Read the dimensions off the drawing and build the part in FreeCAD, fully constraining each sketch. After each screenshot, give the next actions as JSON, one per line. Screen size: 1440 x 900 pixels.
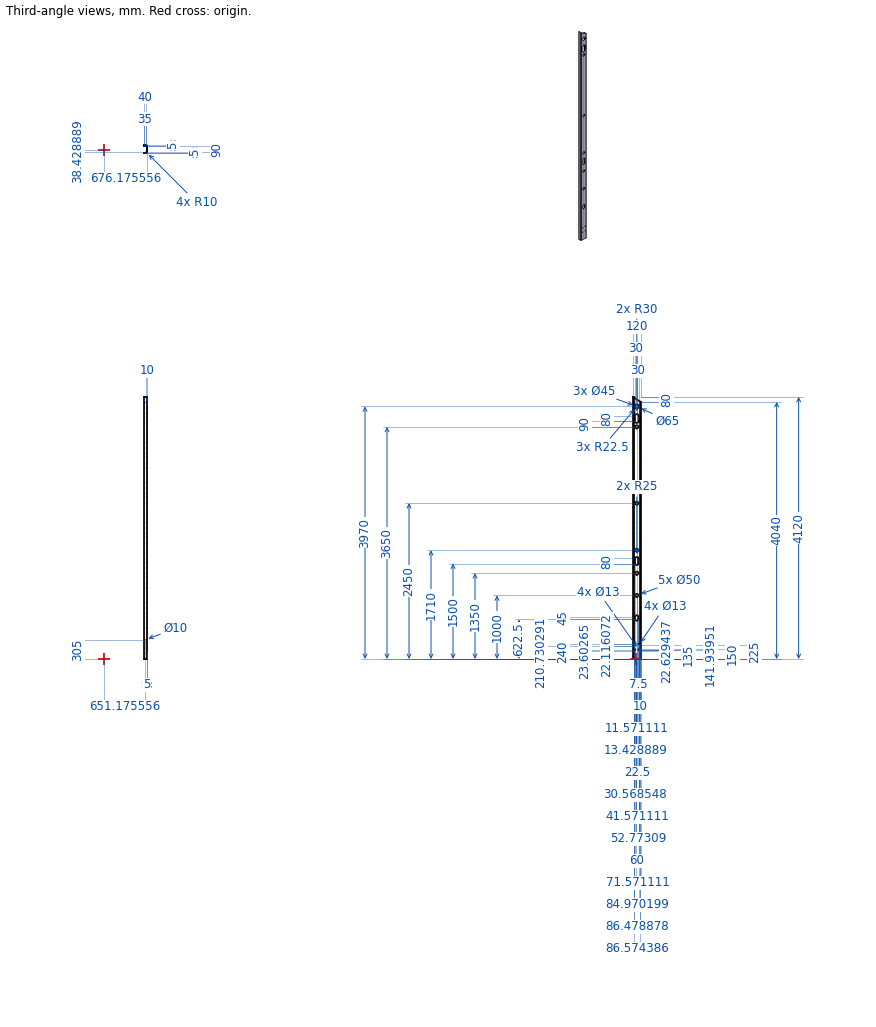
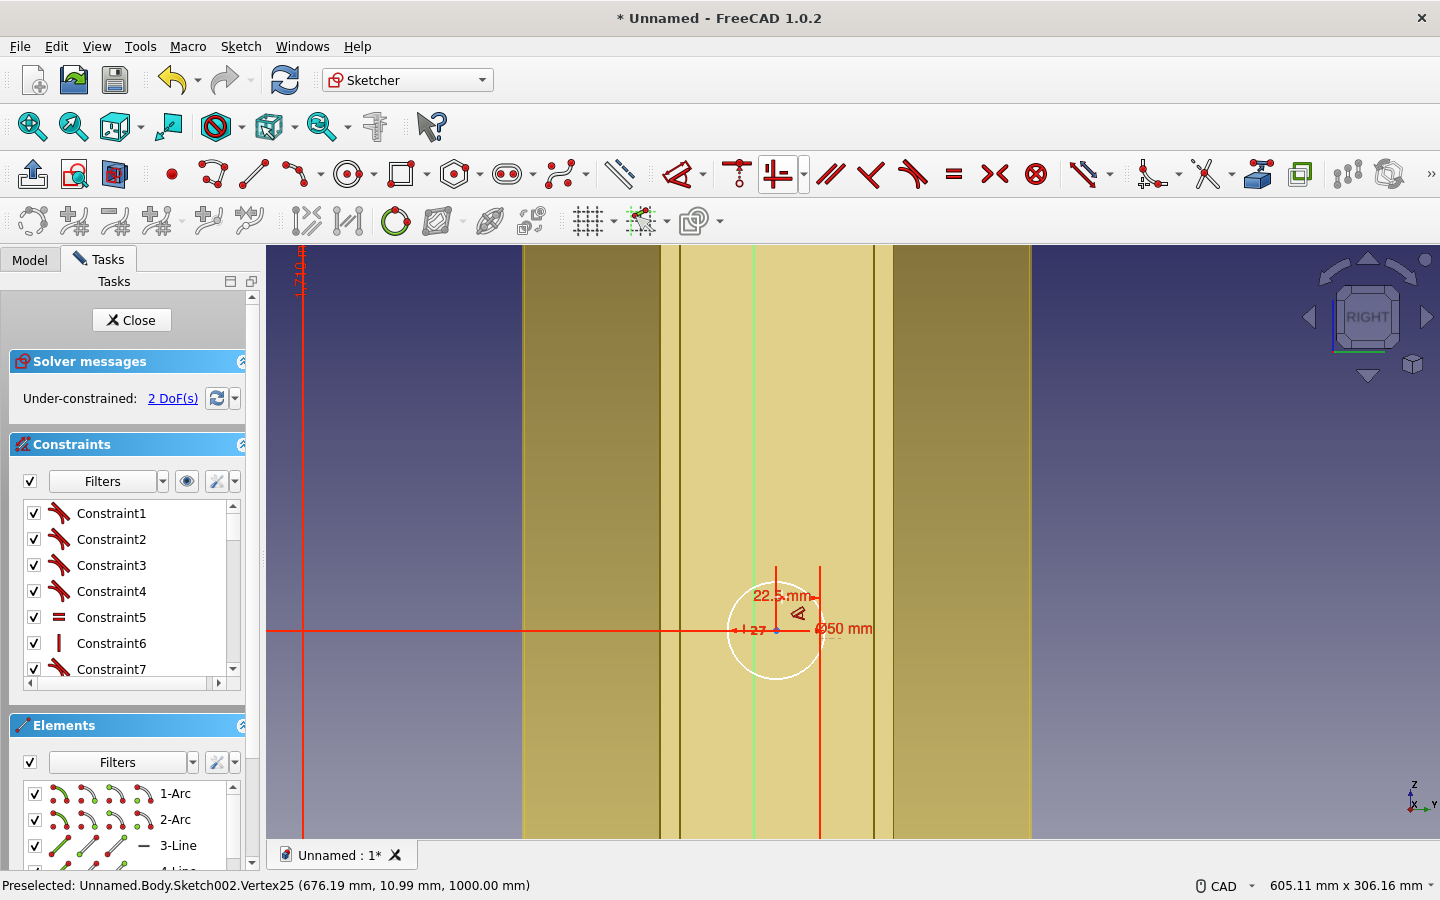
{"action": "scroll", "coordinate": [785, 639], "scroll_direction": "down", "scroll_amount": 15}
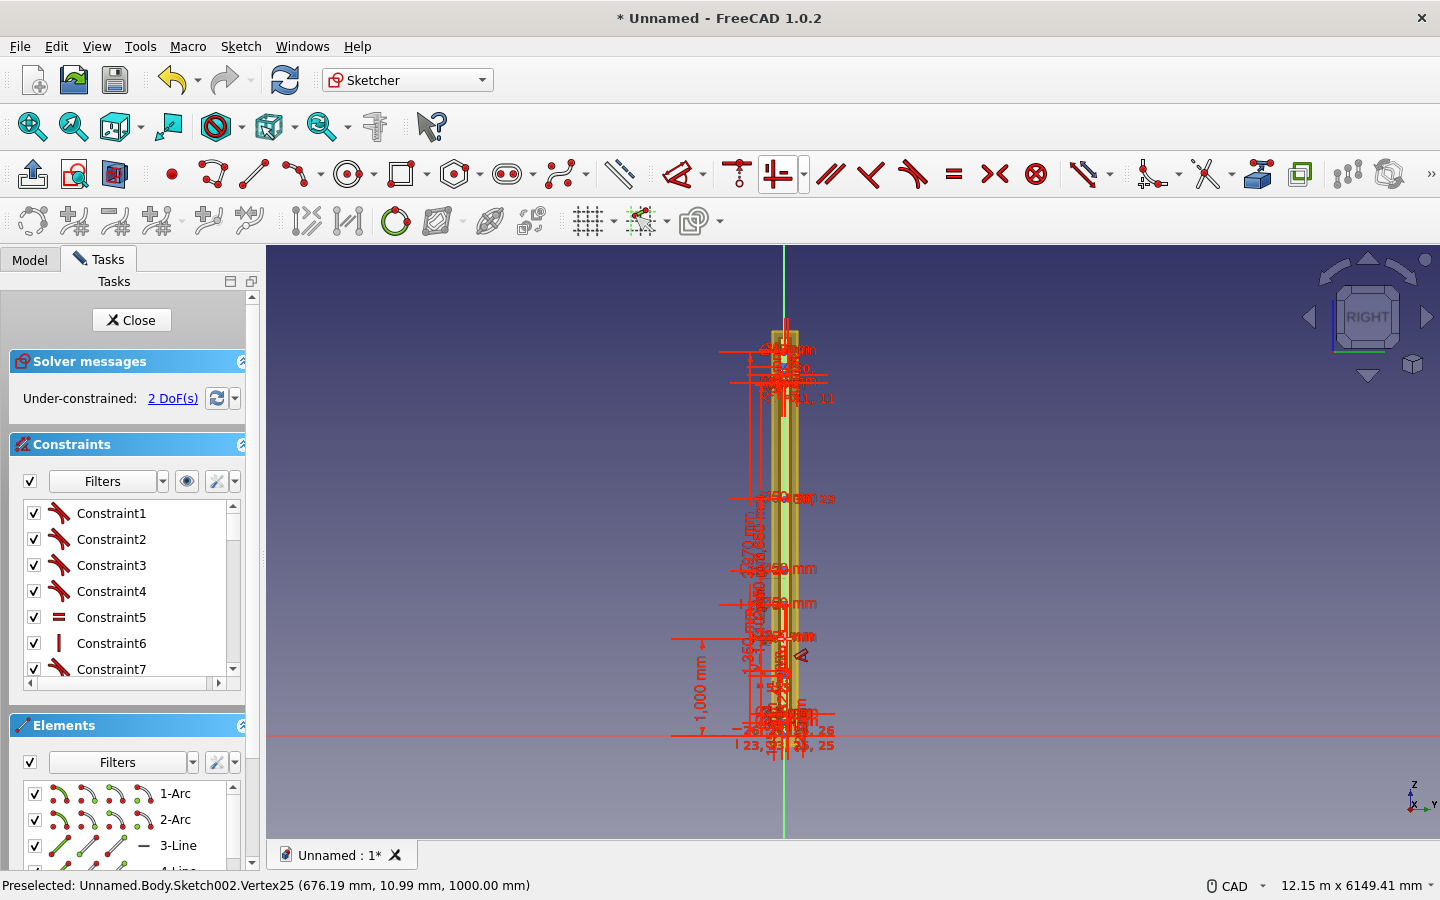
{"action": "scroll", "coordinate": [783, 676], "scroll_direction": "up", "scroll_amount": 9}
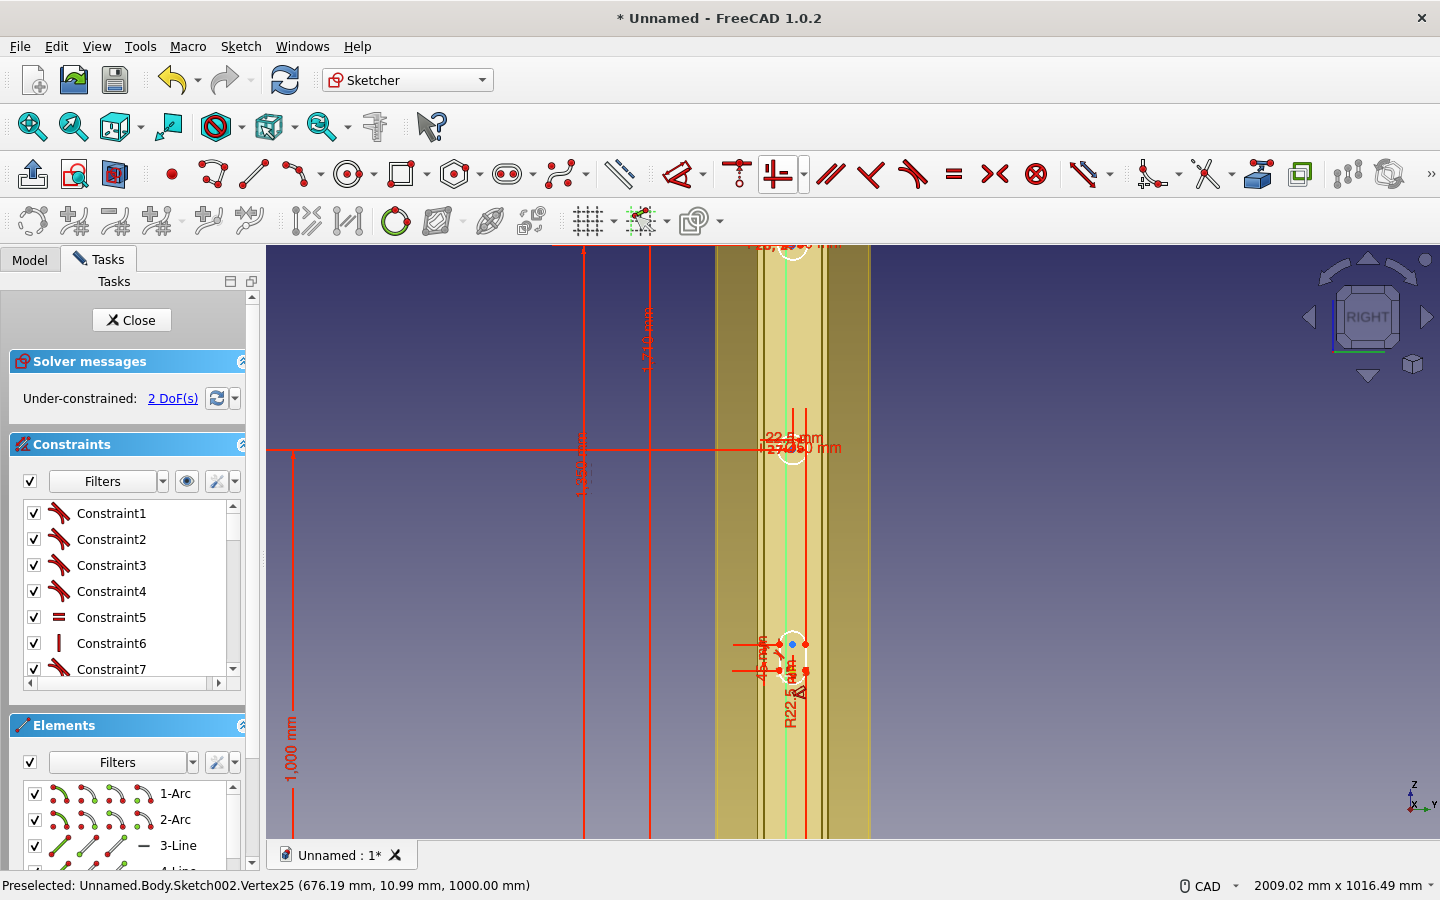
{"action": "left_click", "coordinate": [780, 671]}
{"action": "left_click", "coordinate": [746, 741]}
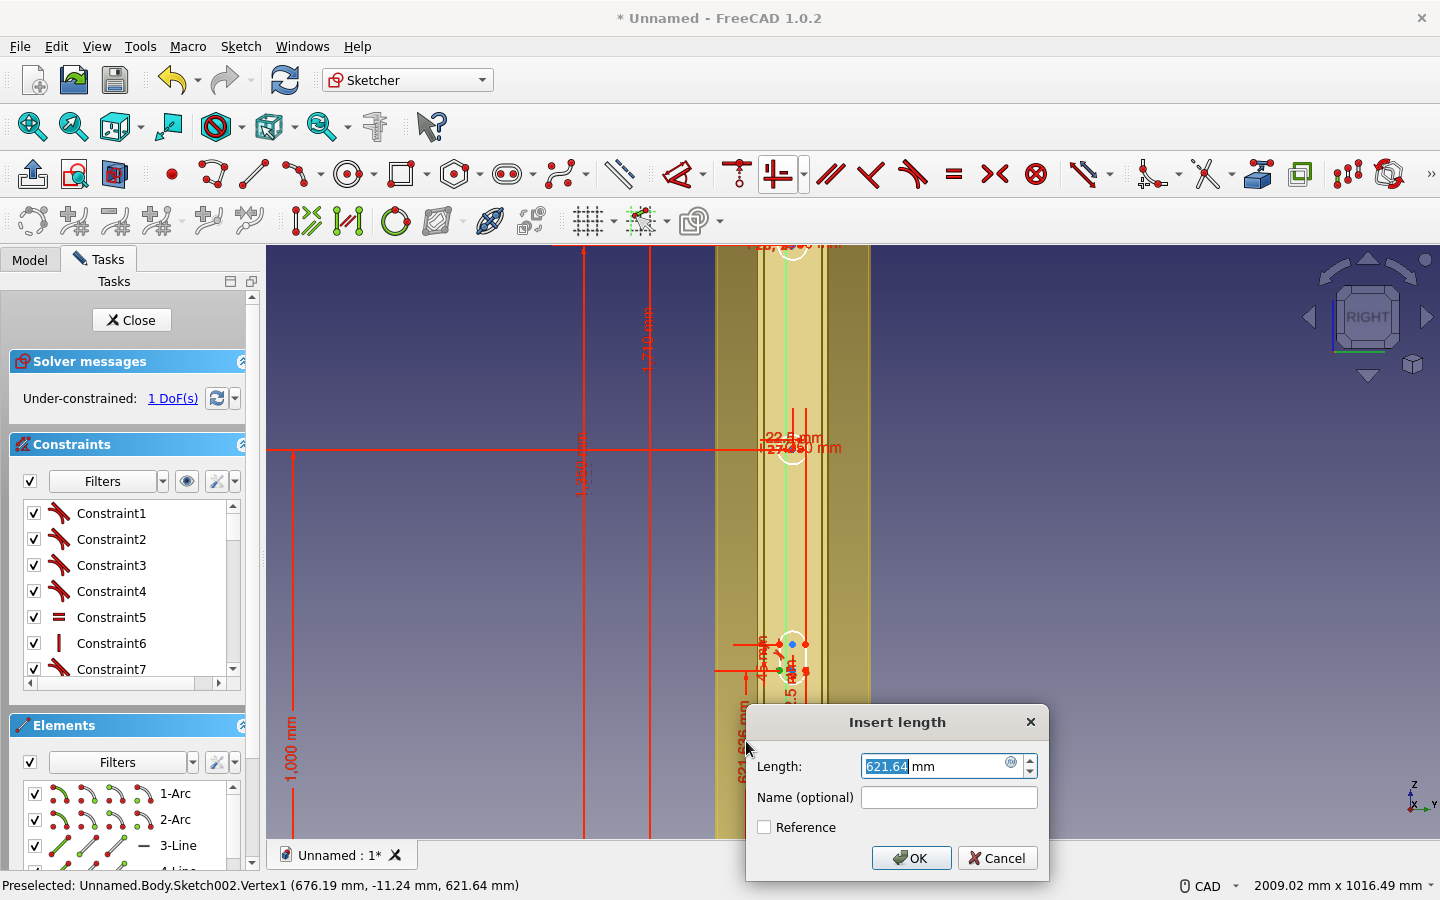
{"action": "type", "text": "622.5"}
{"action": "key", "text": "Return"}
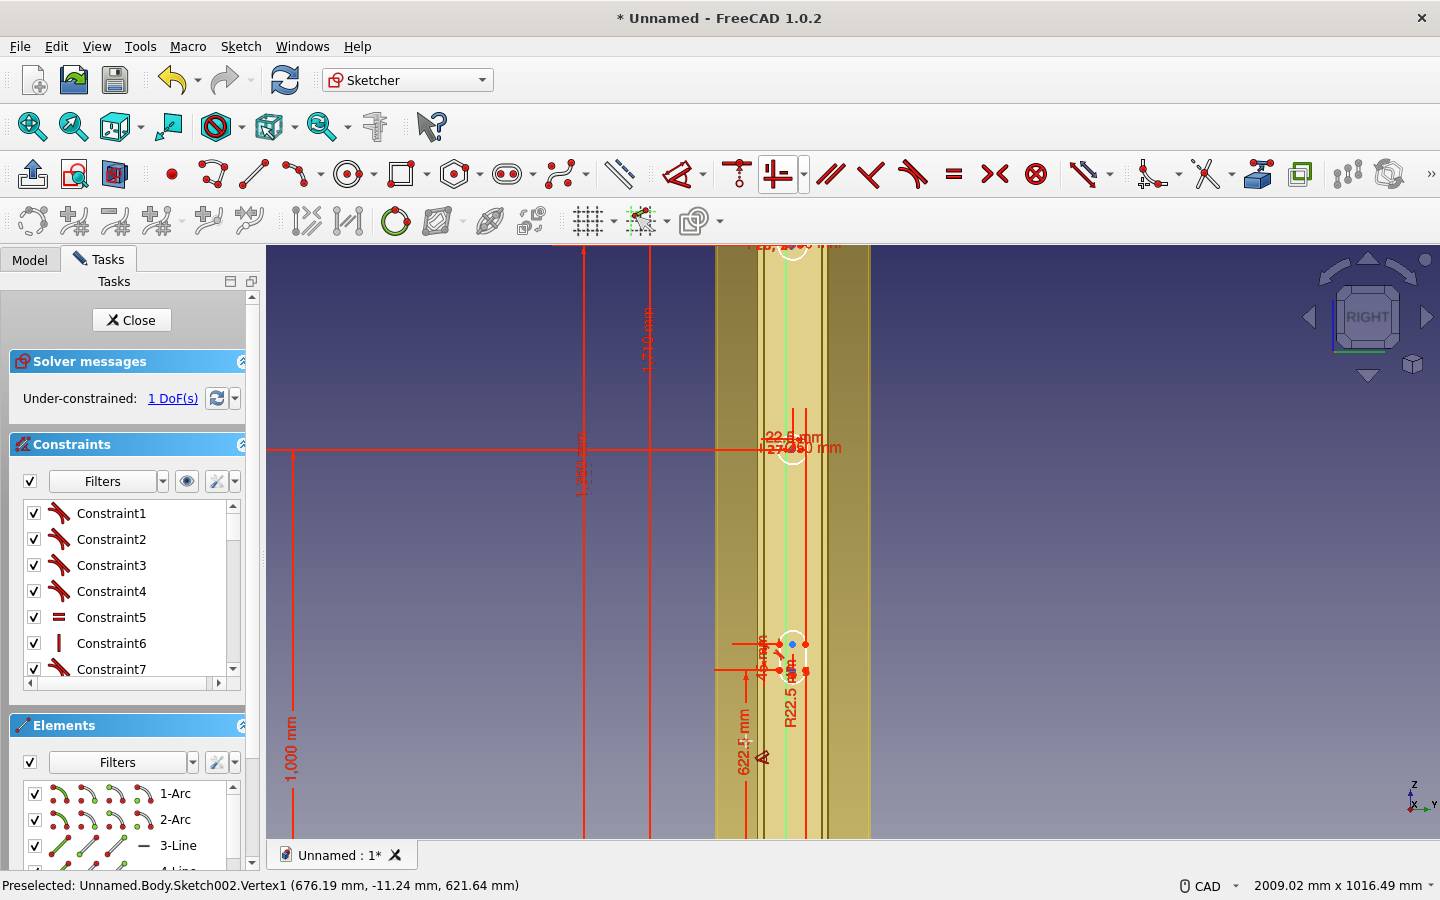
{"action": "scroll", "coordinate": [783, 676], "scroll_direction": "down", "scroll_amount": 9}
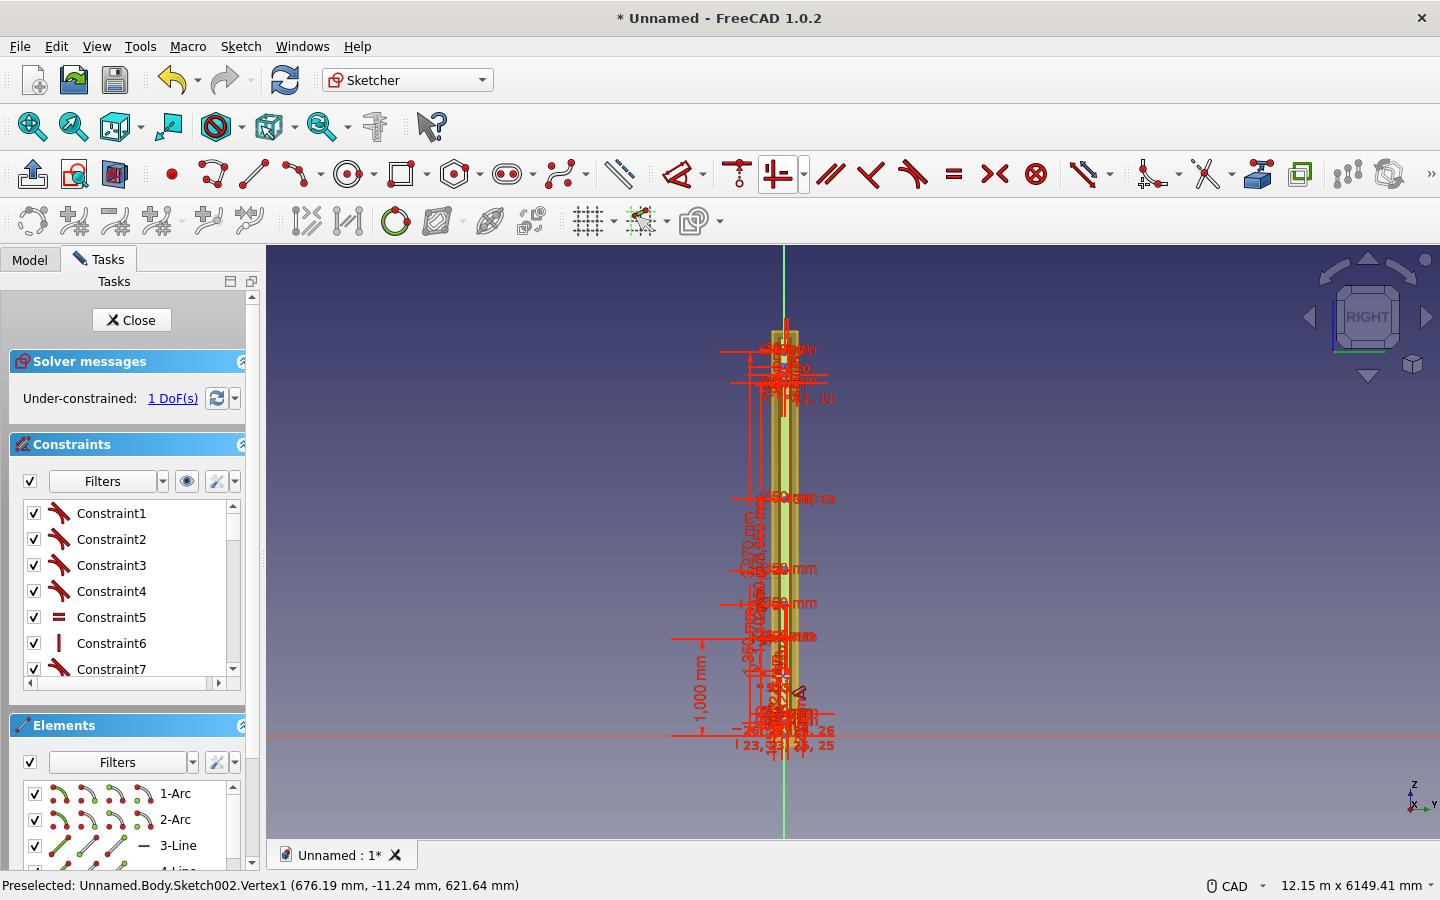
{"action": "scroll", "coordinate": [788, 714], "scroll_direction": "up", "scroll_amount": 12}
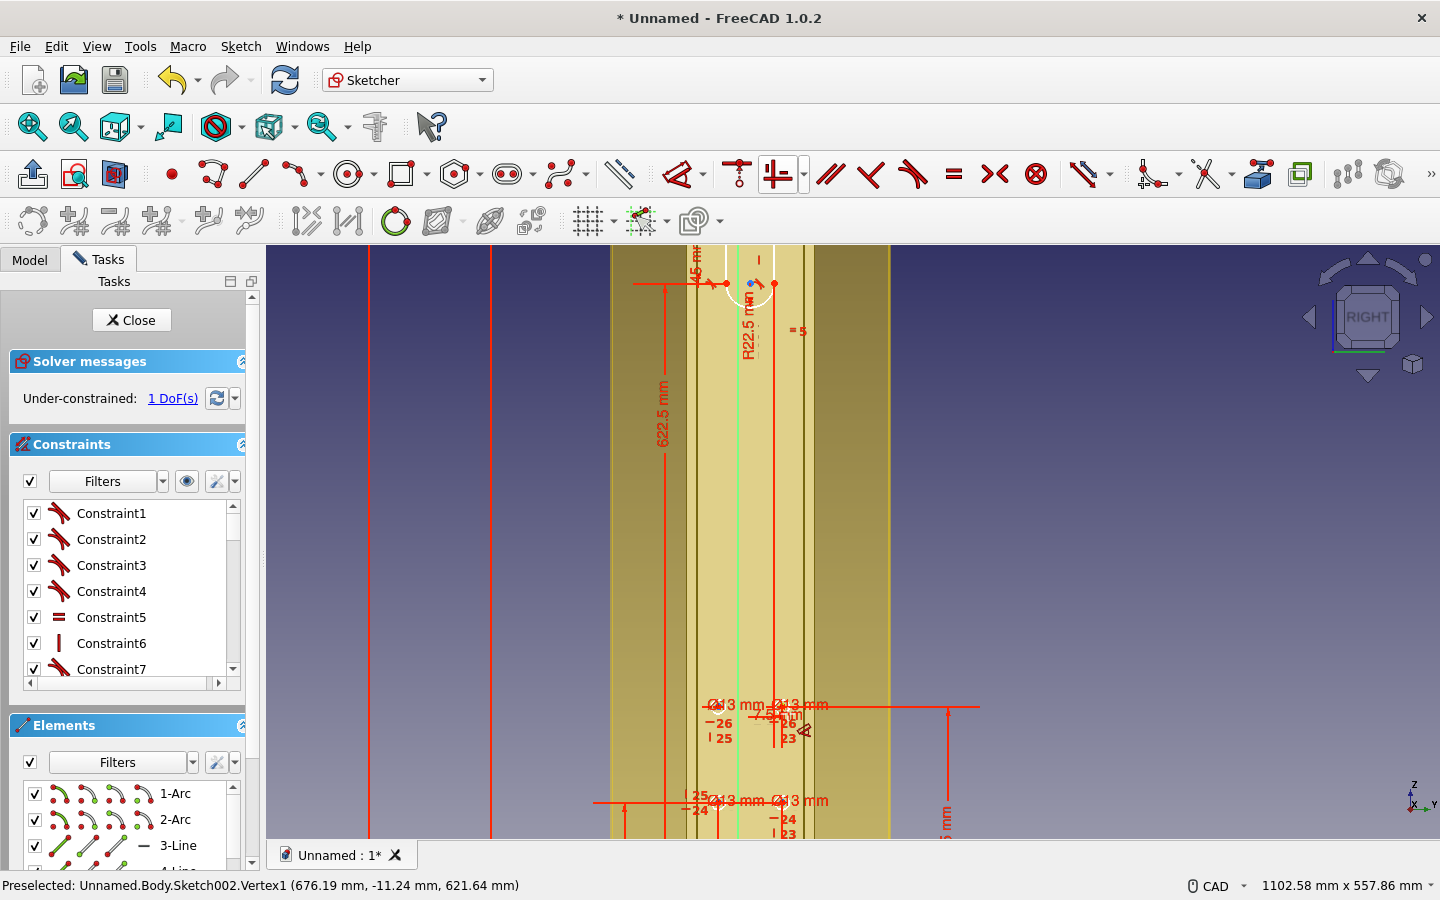
{"action": "left_click", "coordinate": [782, 707]}
{"action": "left_click", "coordinate": [760, 673]}